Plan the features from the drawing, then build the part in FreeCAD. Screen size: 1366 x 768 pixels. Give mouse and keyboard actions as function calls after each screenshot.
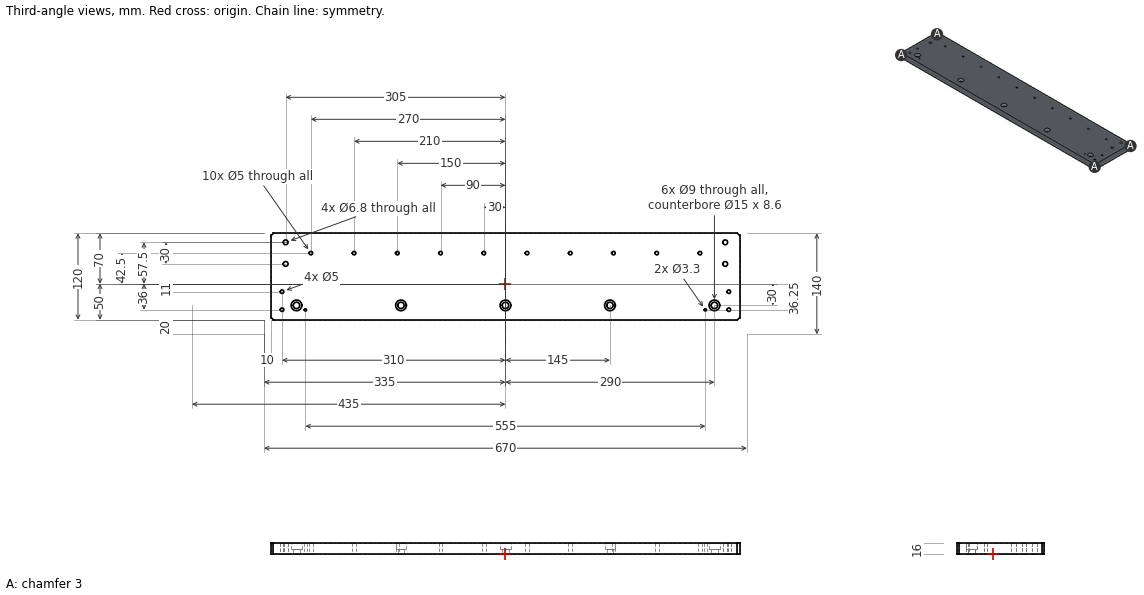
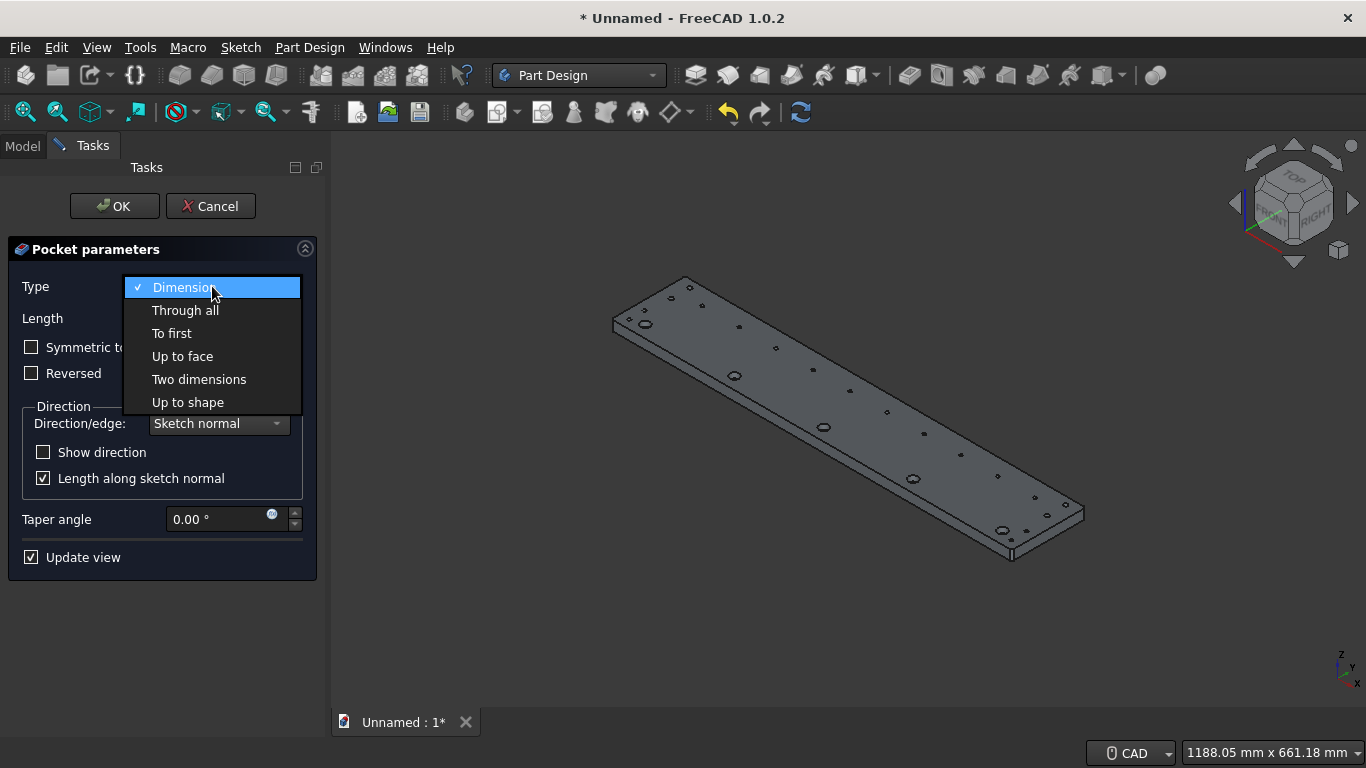
click(212, 310)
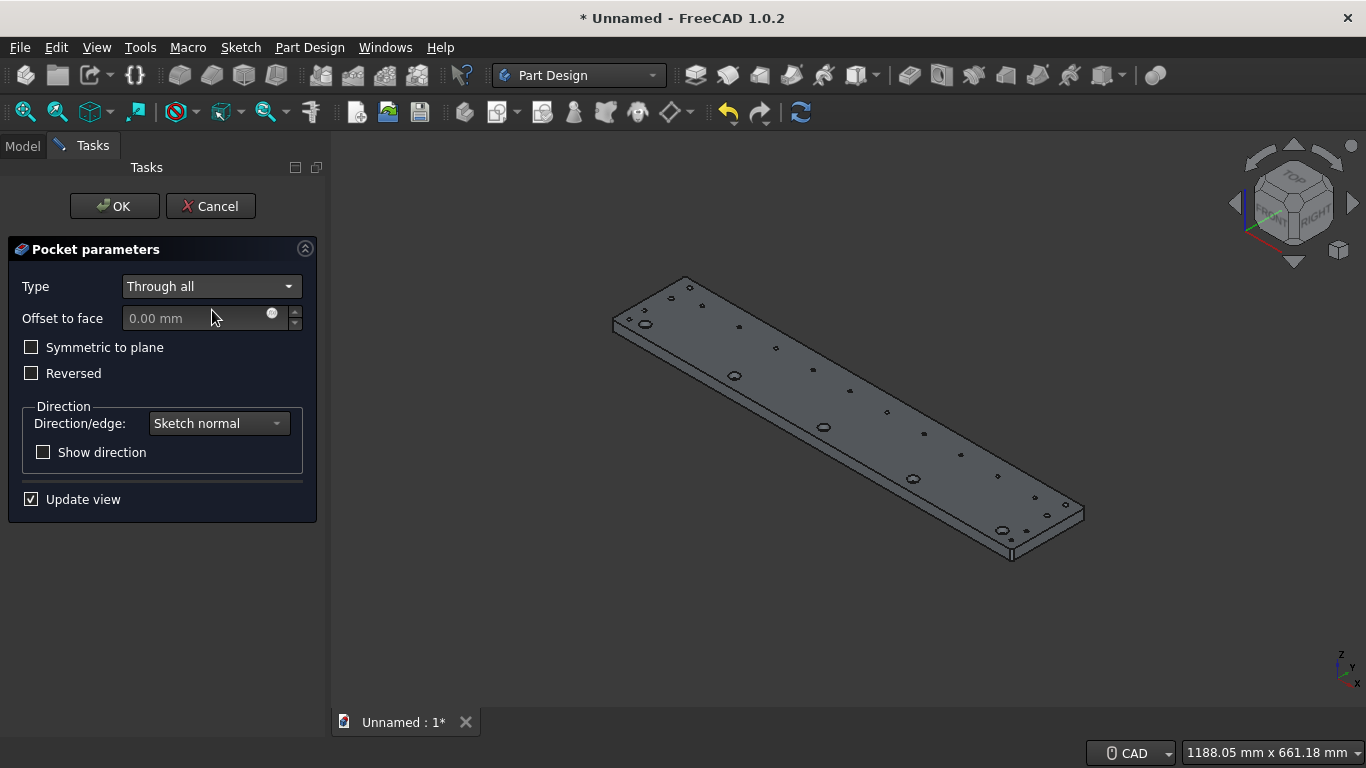
click(115, 206)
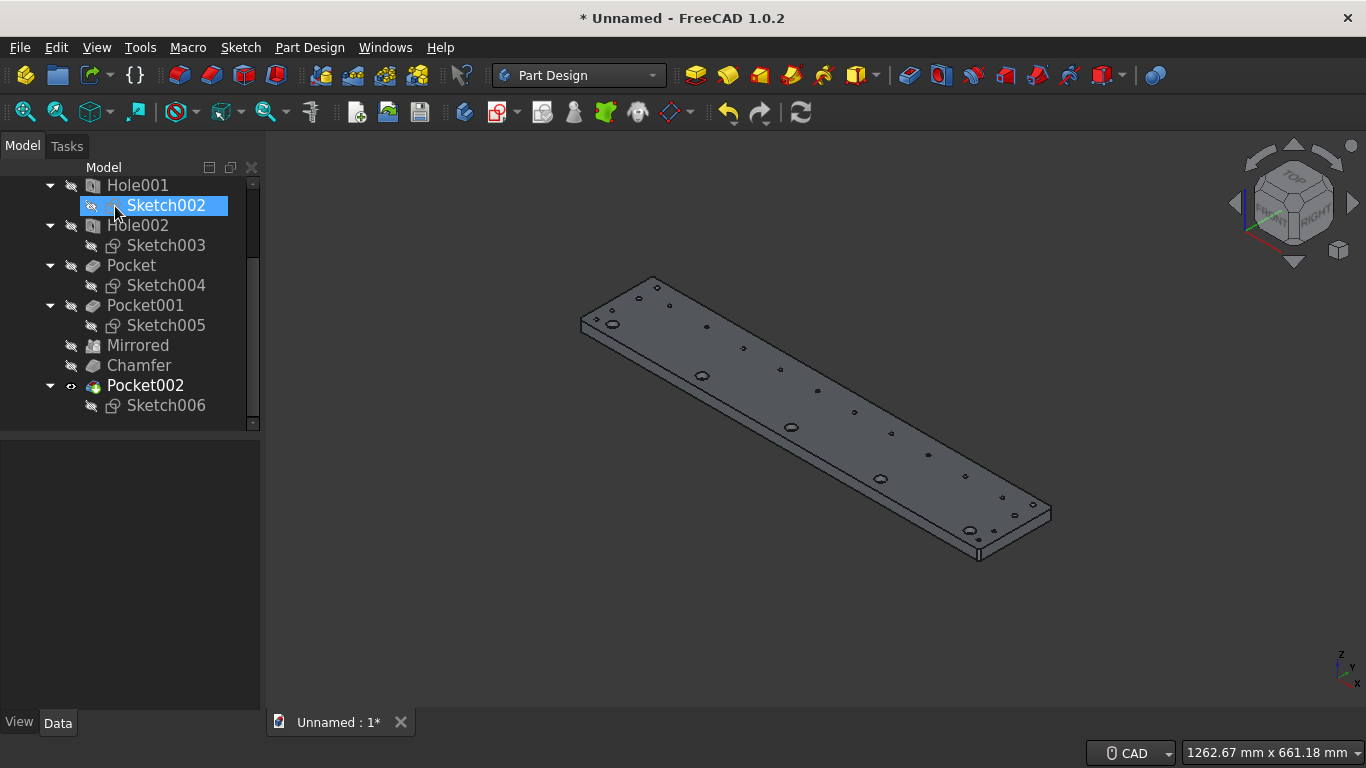
click(863, 451)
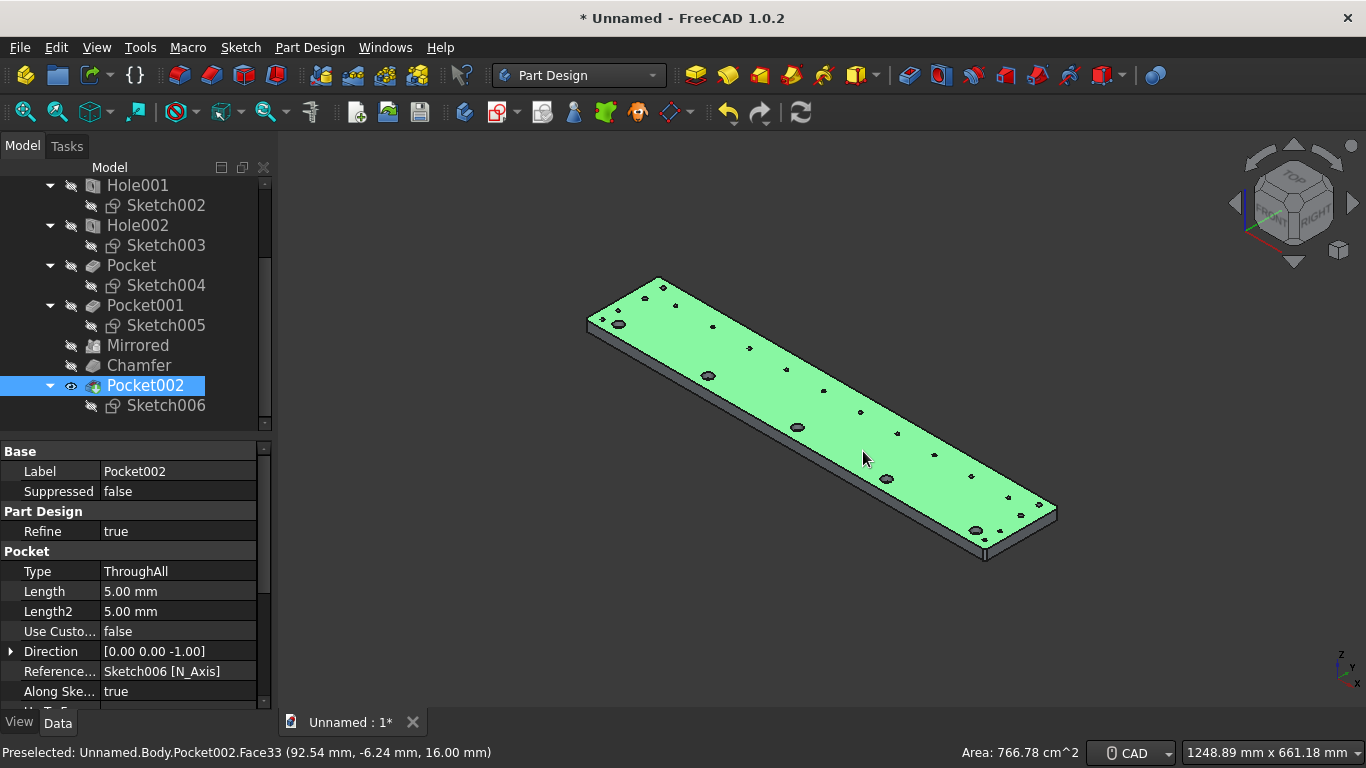
click(498, 112)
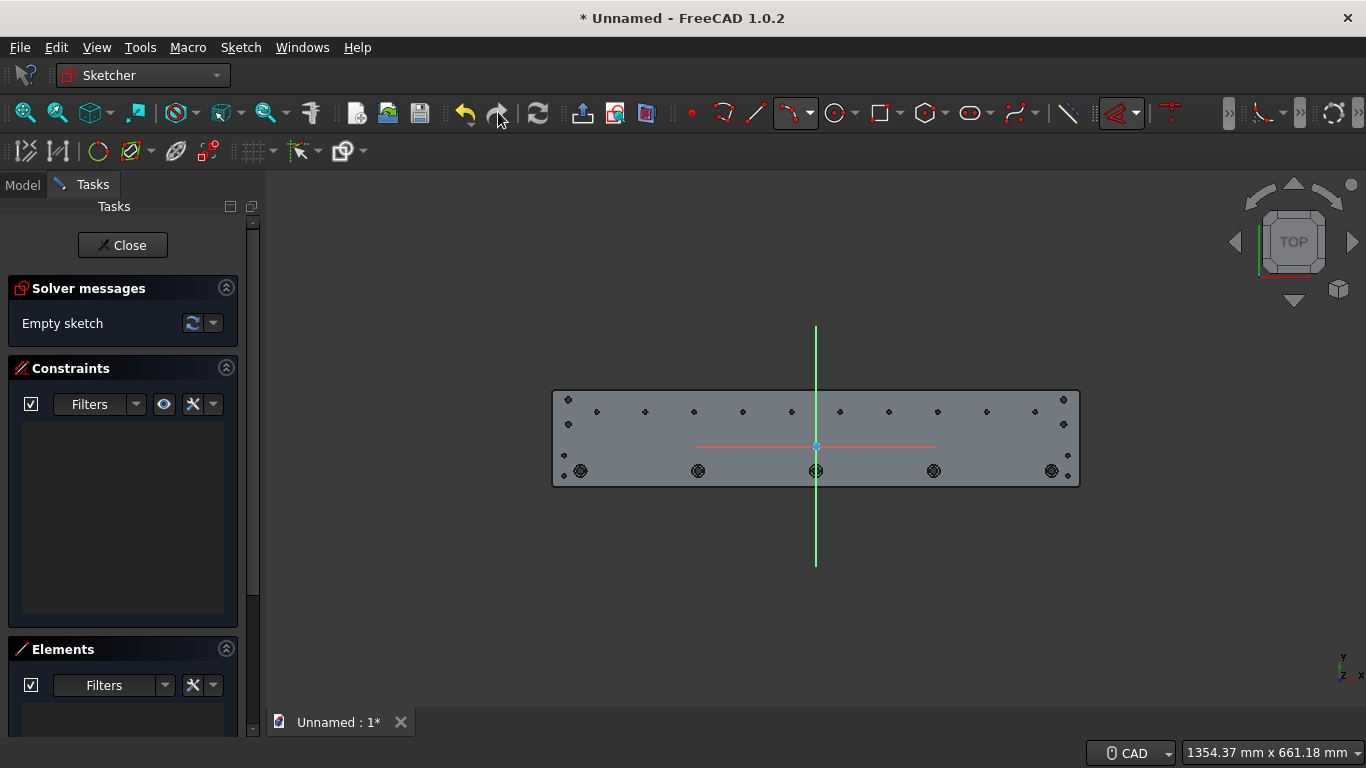
scroll(955, 510, up, 2)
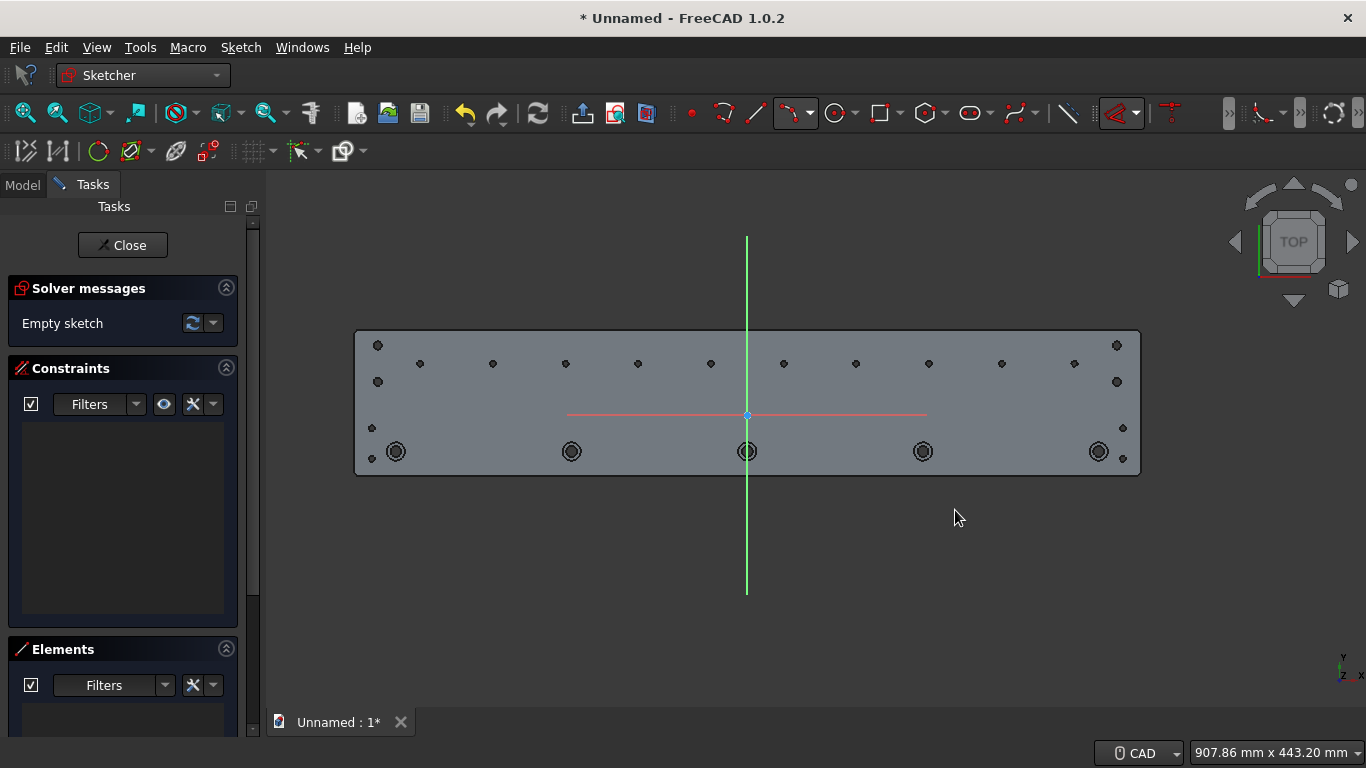
click(836, 114)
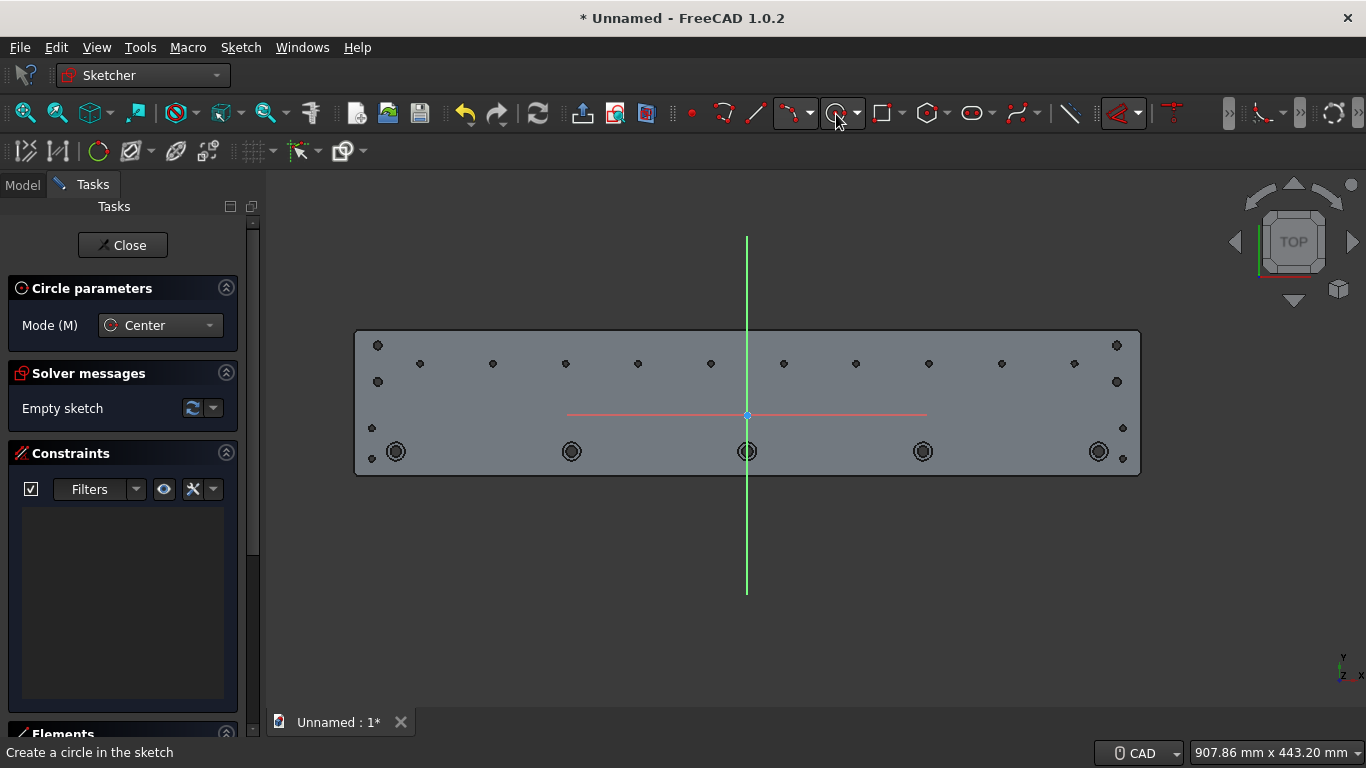
scroll(1084, 459, up, 13)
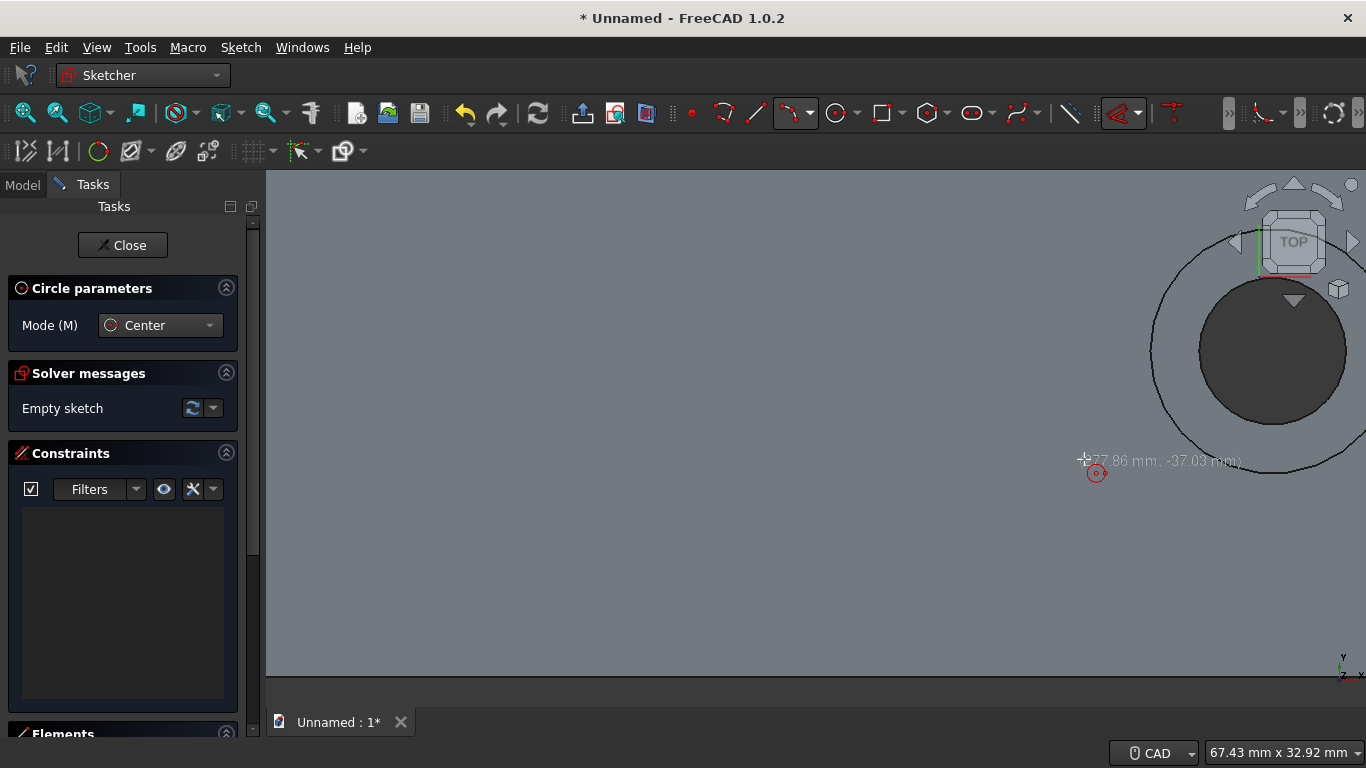
scroll(1085, 460, down, 13)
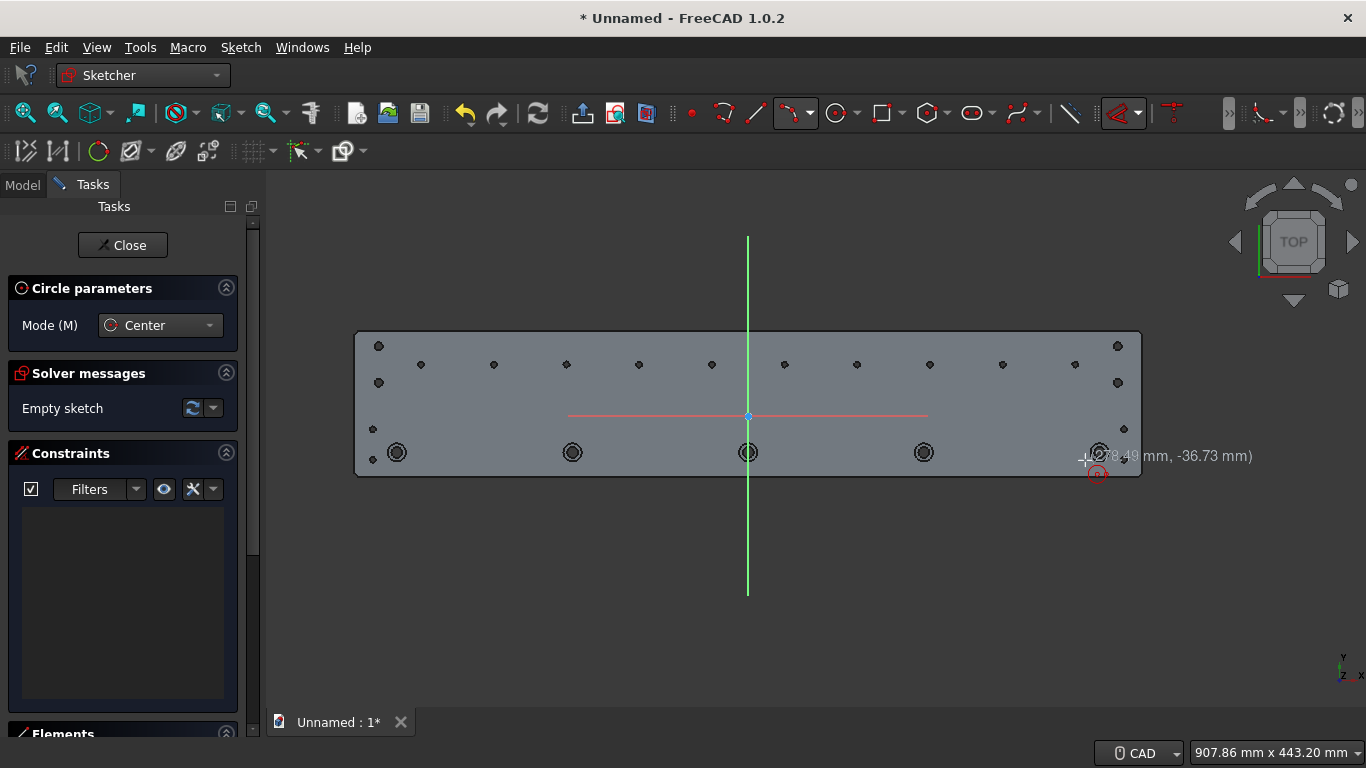
click(1084, 460)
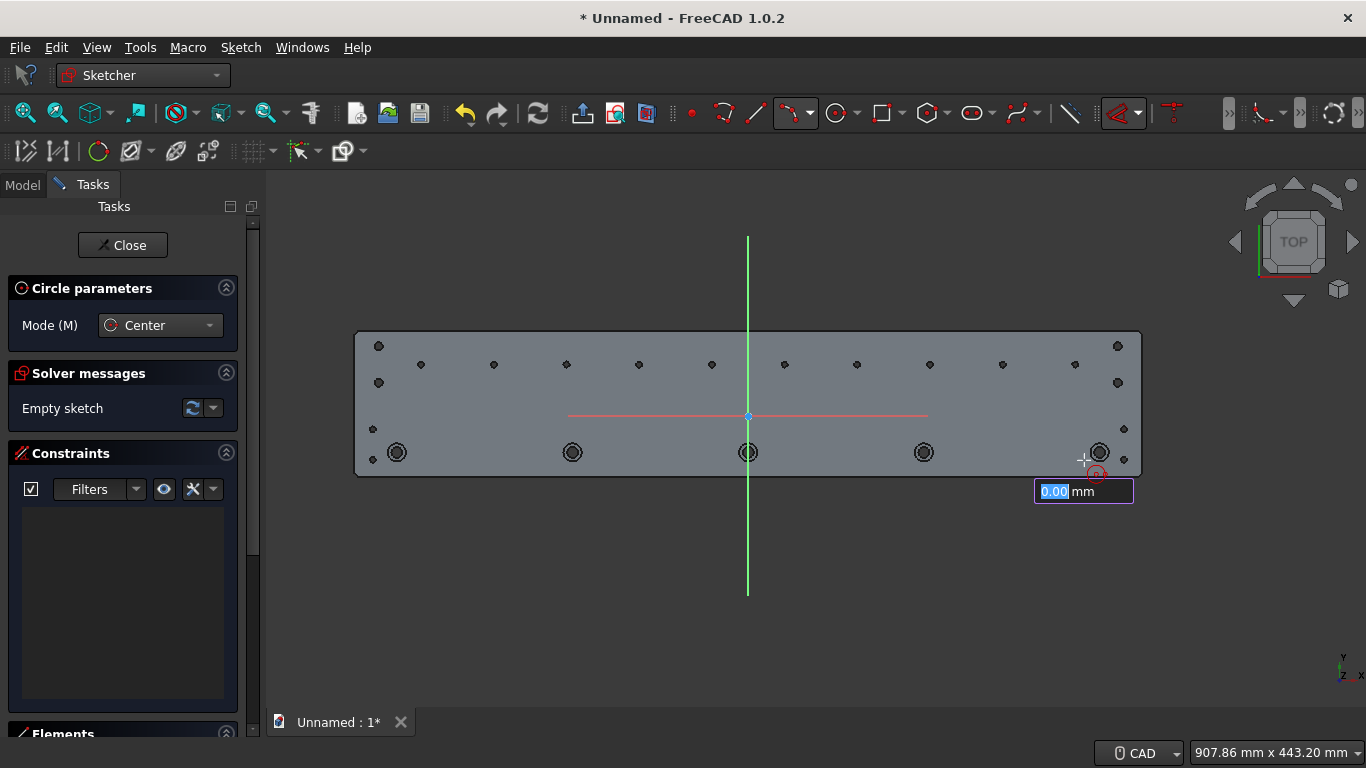
scroll(1086, 459, up, 11)